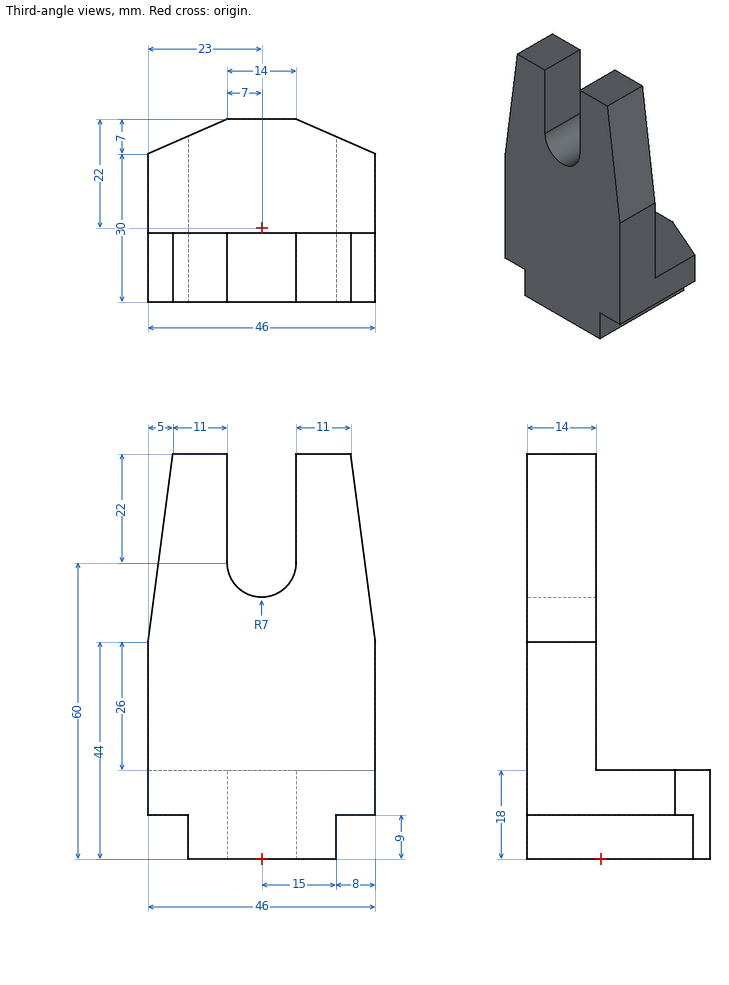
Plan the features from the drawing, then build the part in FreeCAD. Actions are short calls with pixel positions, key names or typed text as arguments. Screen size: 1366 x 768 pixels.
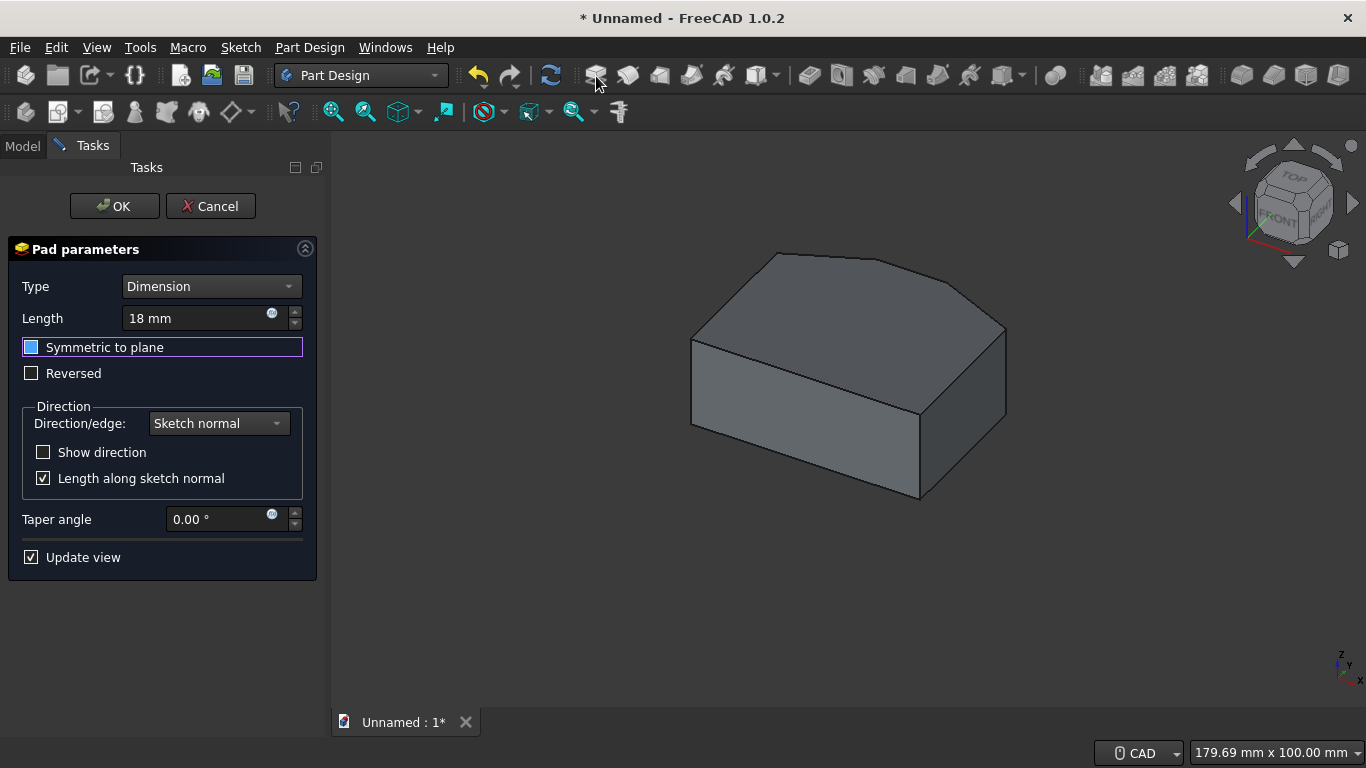
click(115, 206)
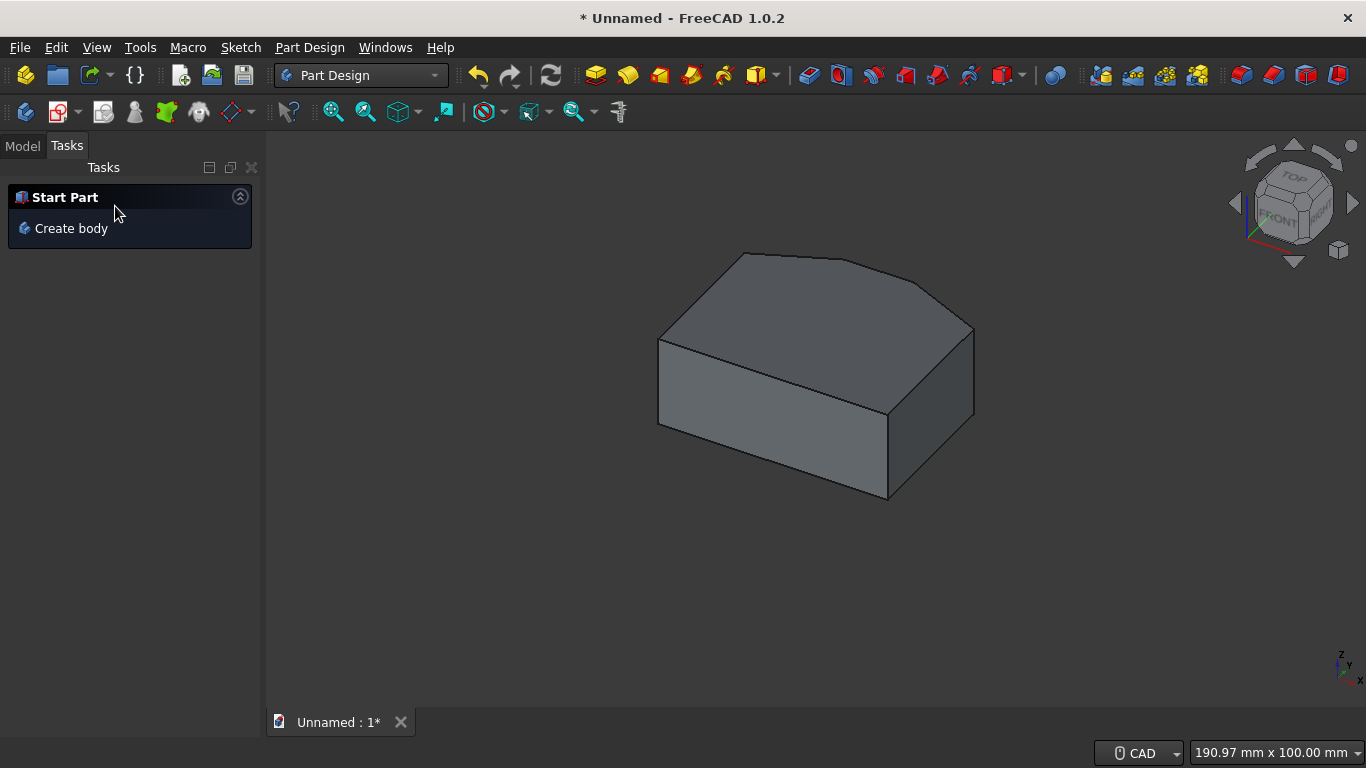
click(838, 440)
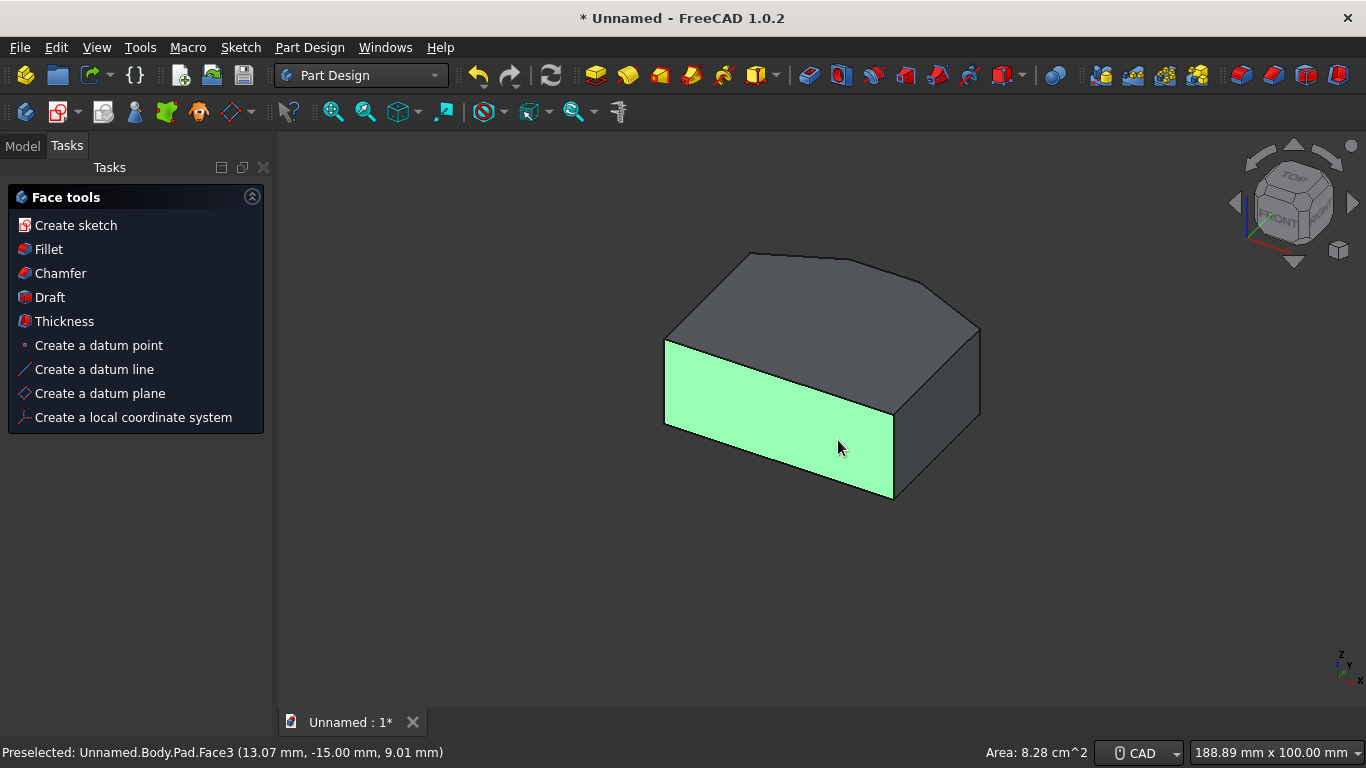
click(58, 112)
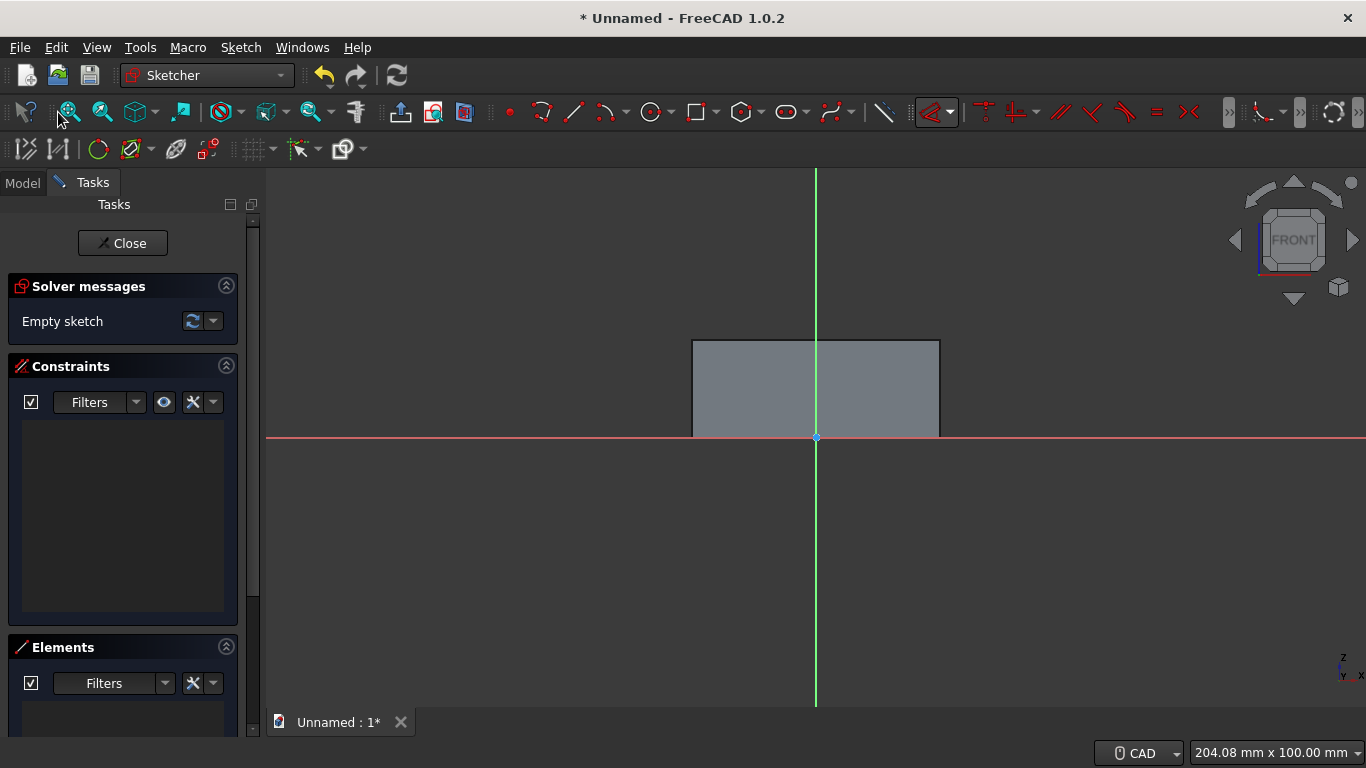
scroll(664, 679, down, 3)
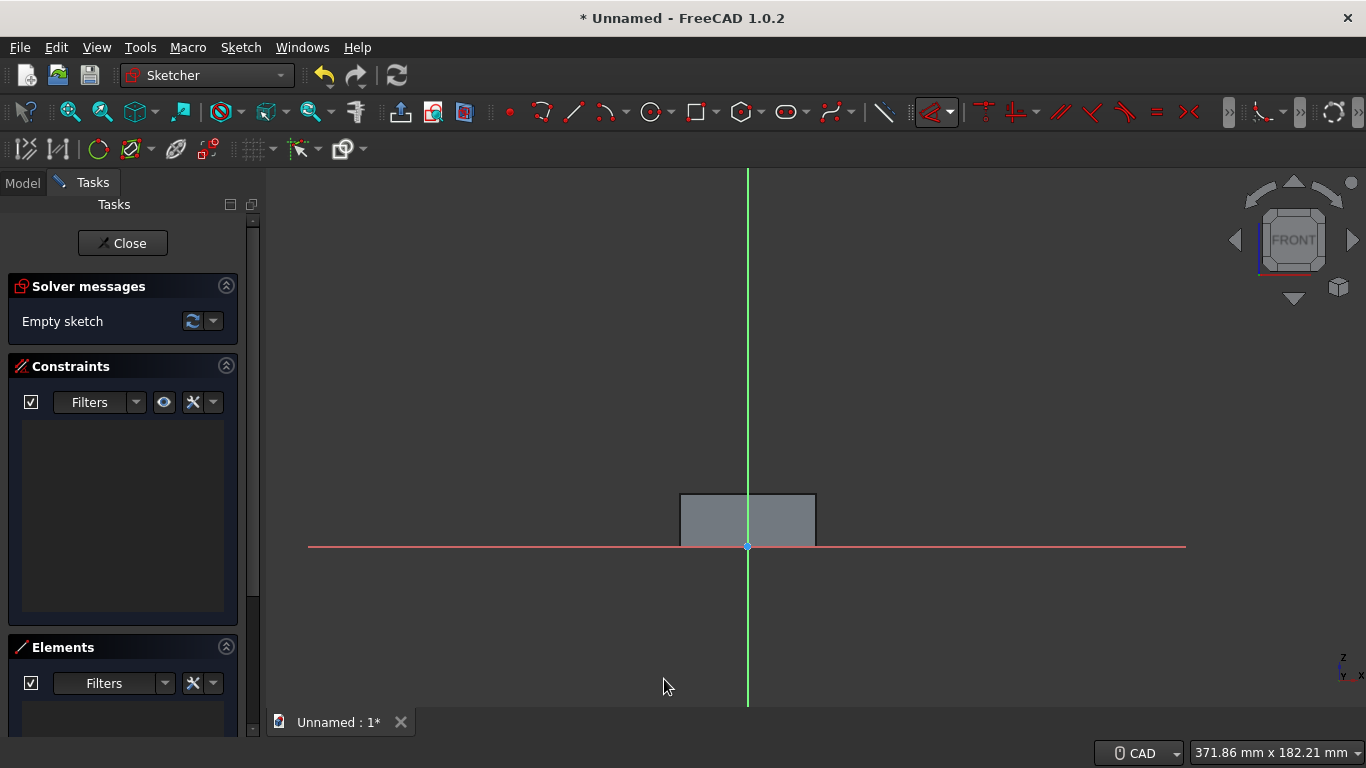
scroll(748, 401, up, 2)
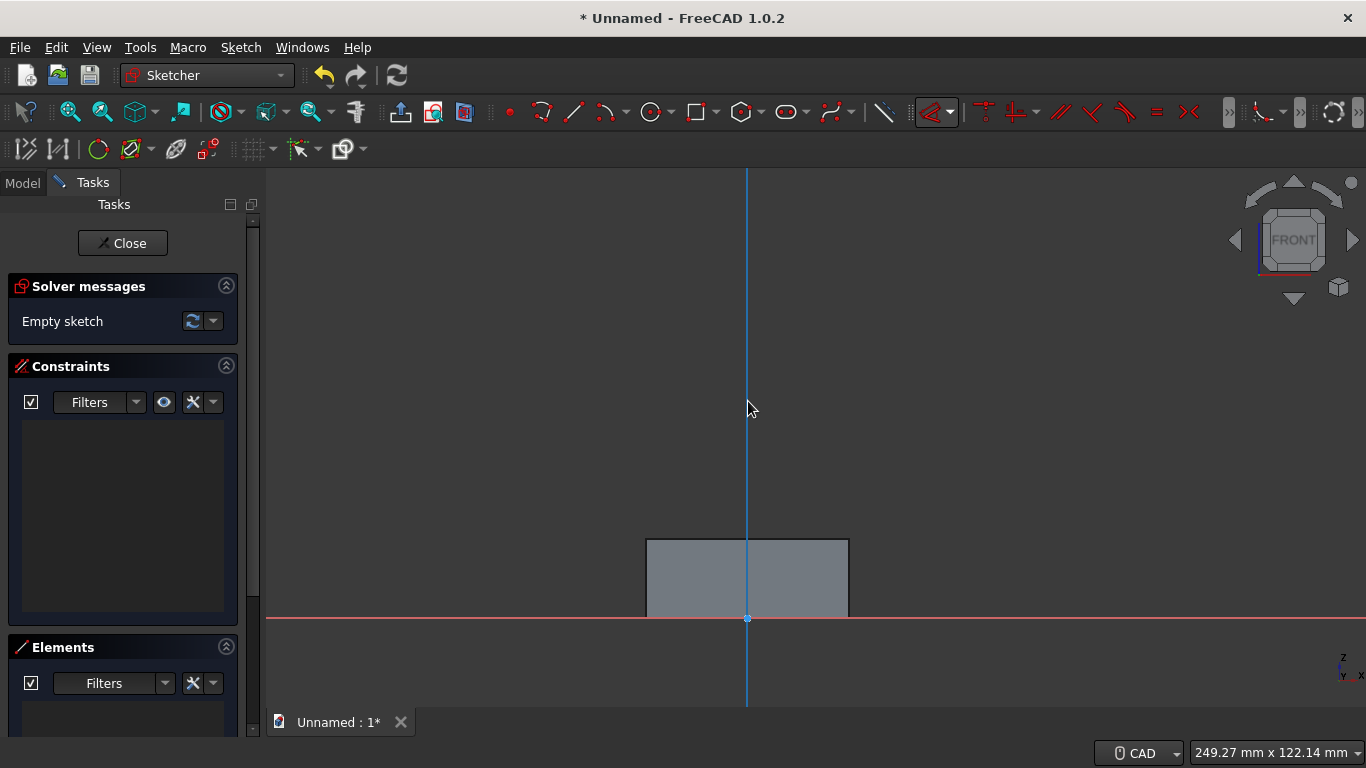
click(542, 112)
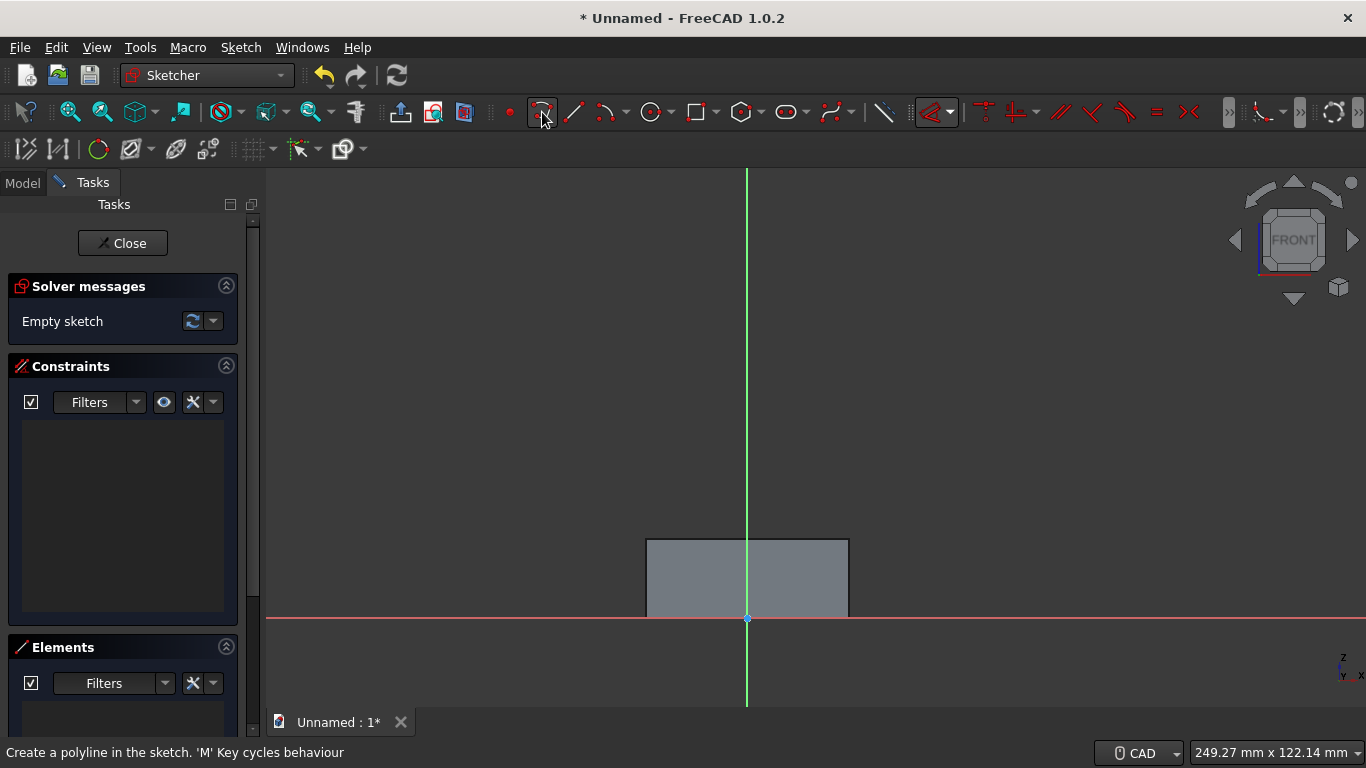
click(716, 354)
click(716, 257)
click(668, 257)
click(646, 424)
click(646, 539)
click(849, 539)
click(849, 424)
click(827, 257)
click(778, 257)
click(778, 354)
right_click(778, 354)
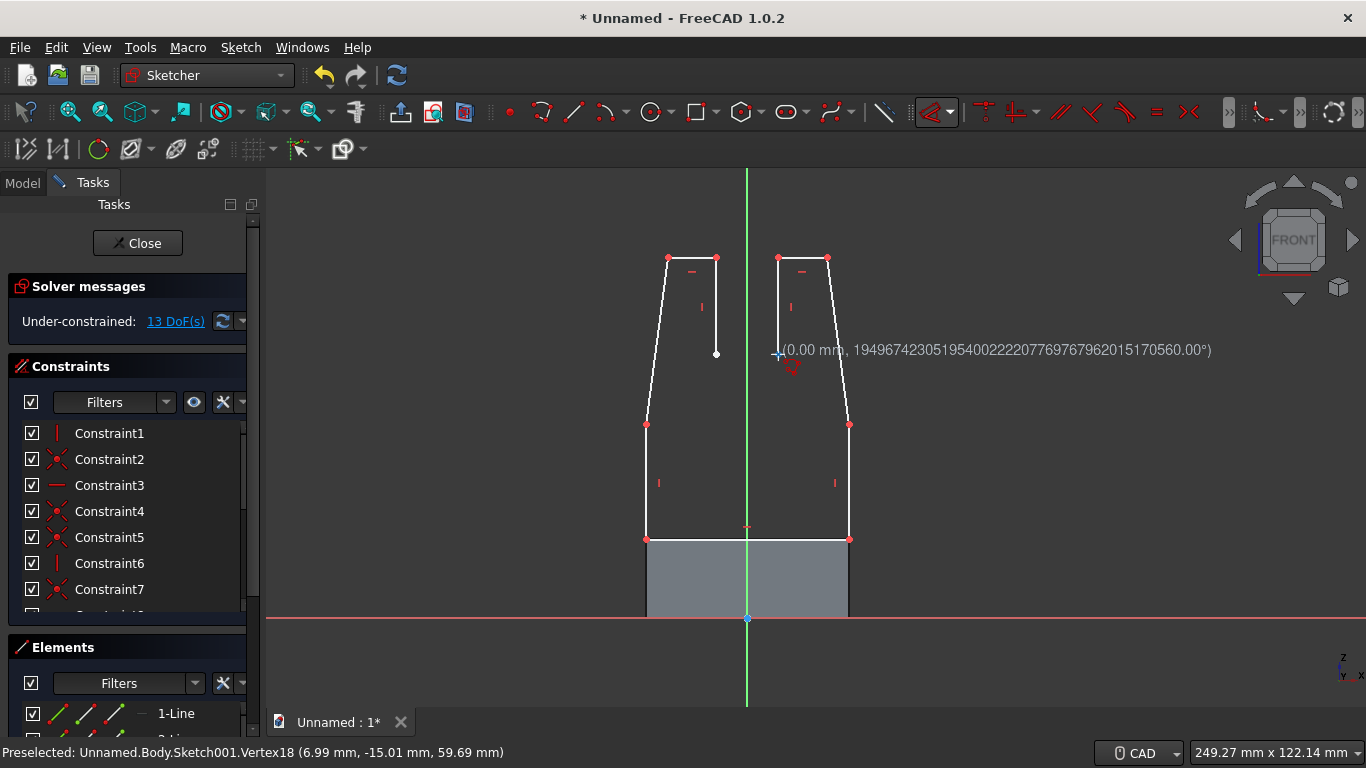
click(628, 112)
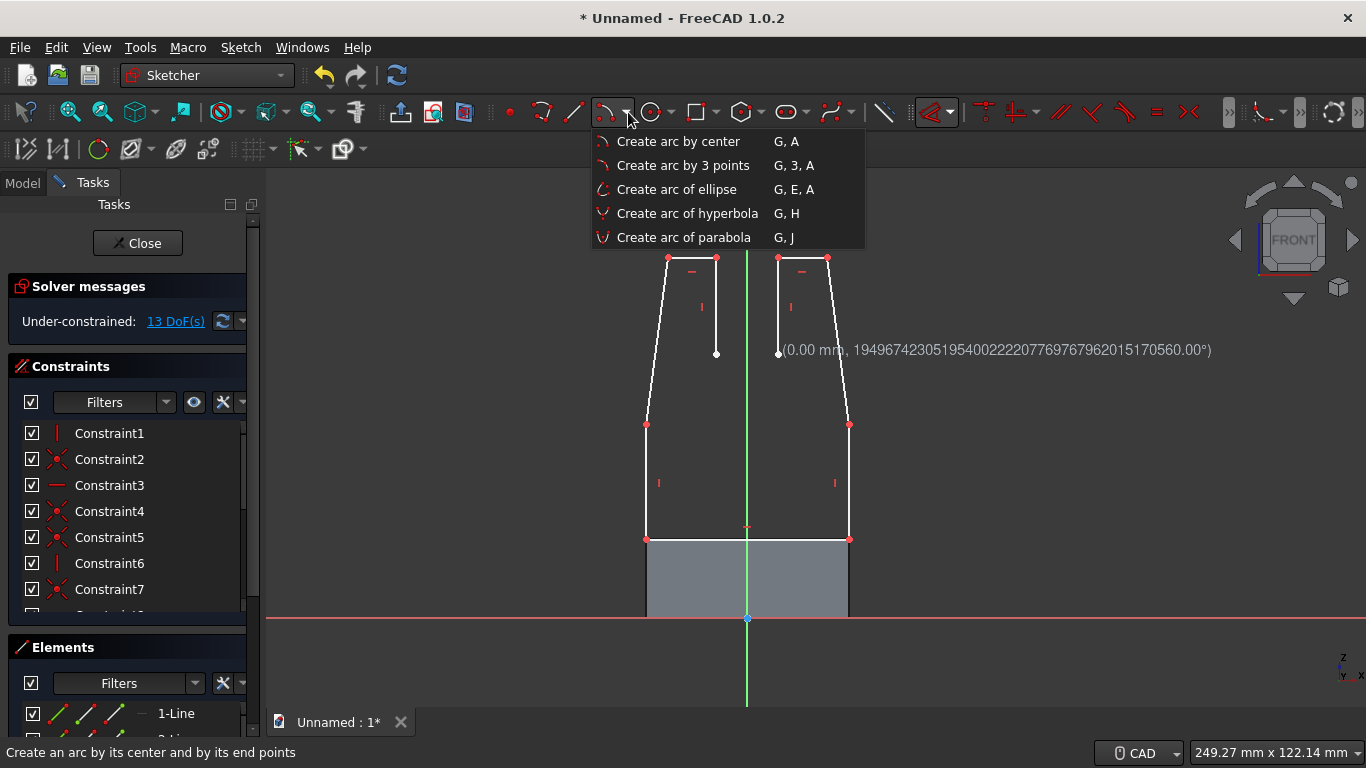
click(728, 165)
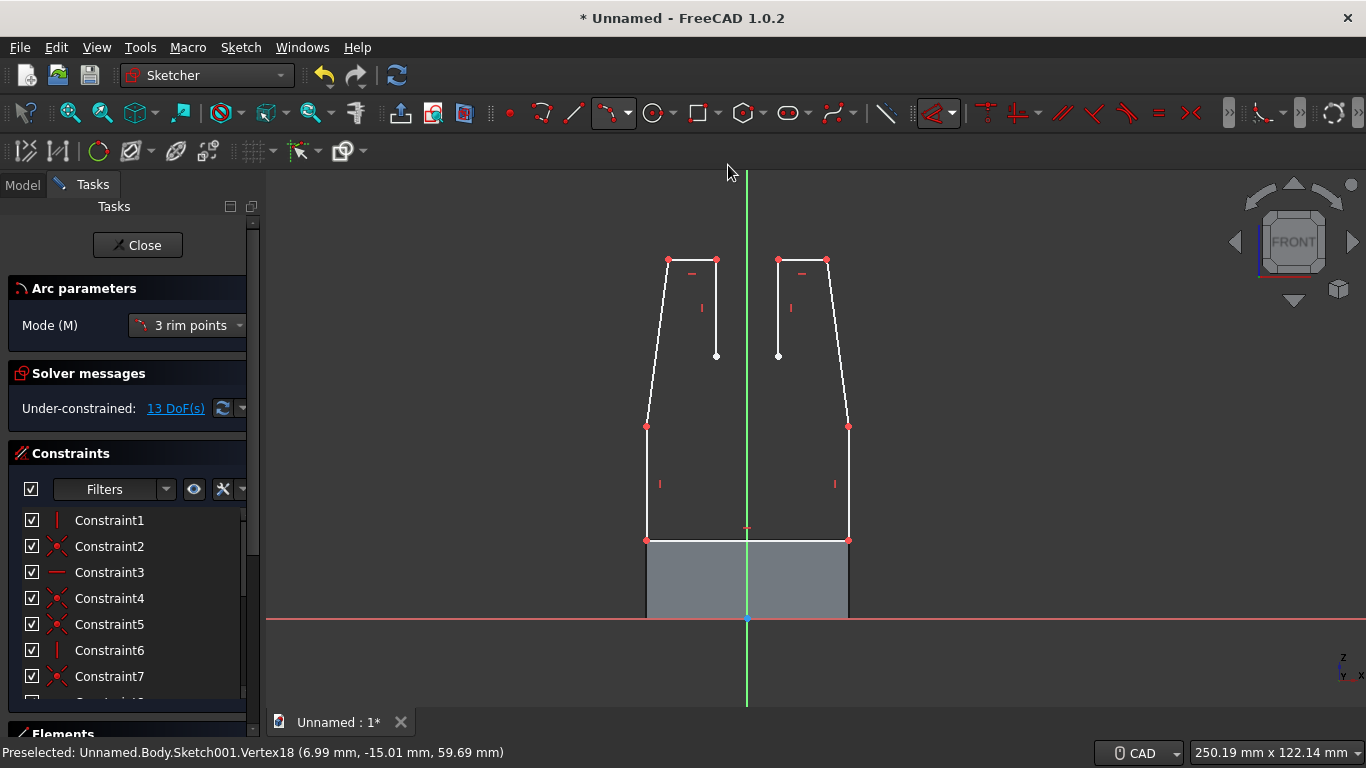
click(778, 356)
click(716, 356)
click(729, 380)
key(Escape)